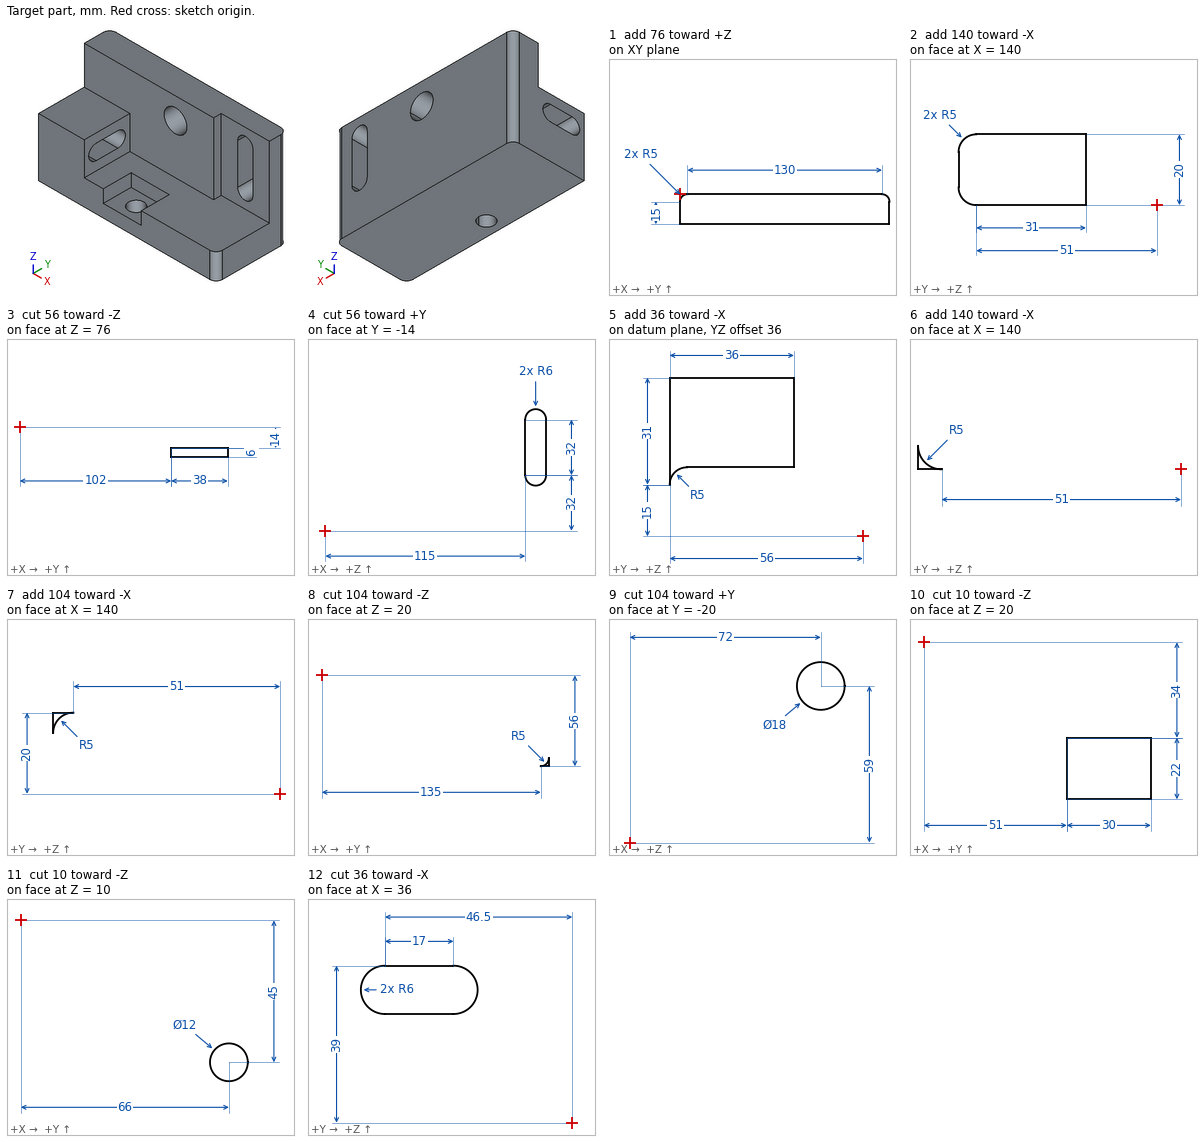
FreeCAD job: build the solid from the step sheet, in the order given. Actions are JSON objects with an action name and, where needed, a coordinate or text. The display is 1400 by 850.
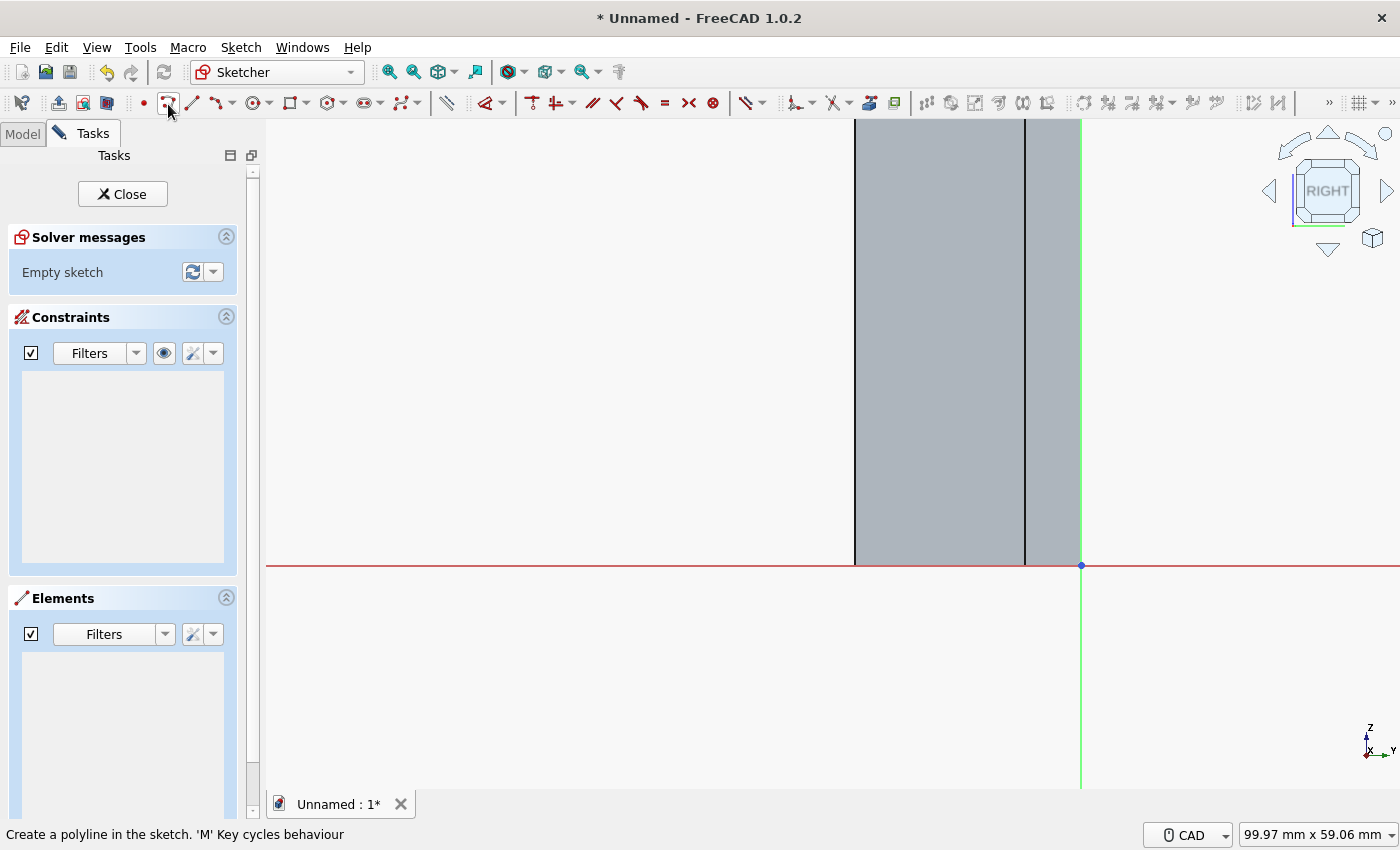
{"action": "left_click", "coordinate": [503, 566]}
{"action": "left_click", "coordinate": [855, 557]}
{"action": "left_click", "coordinate": [855, 339]}
{"action": "left_click", "coordinate": [503, 339]}
{"action": "right_click", "coordinate": [503, 339]}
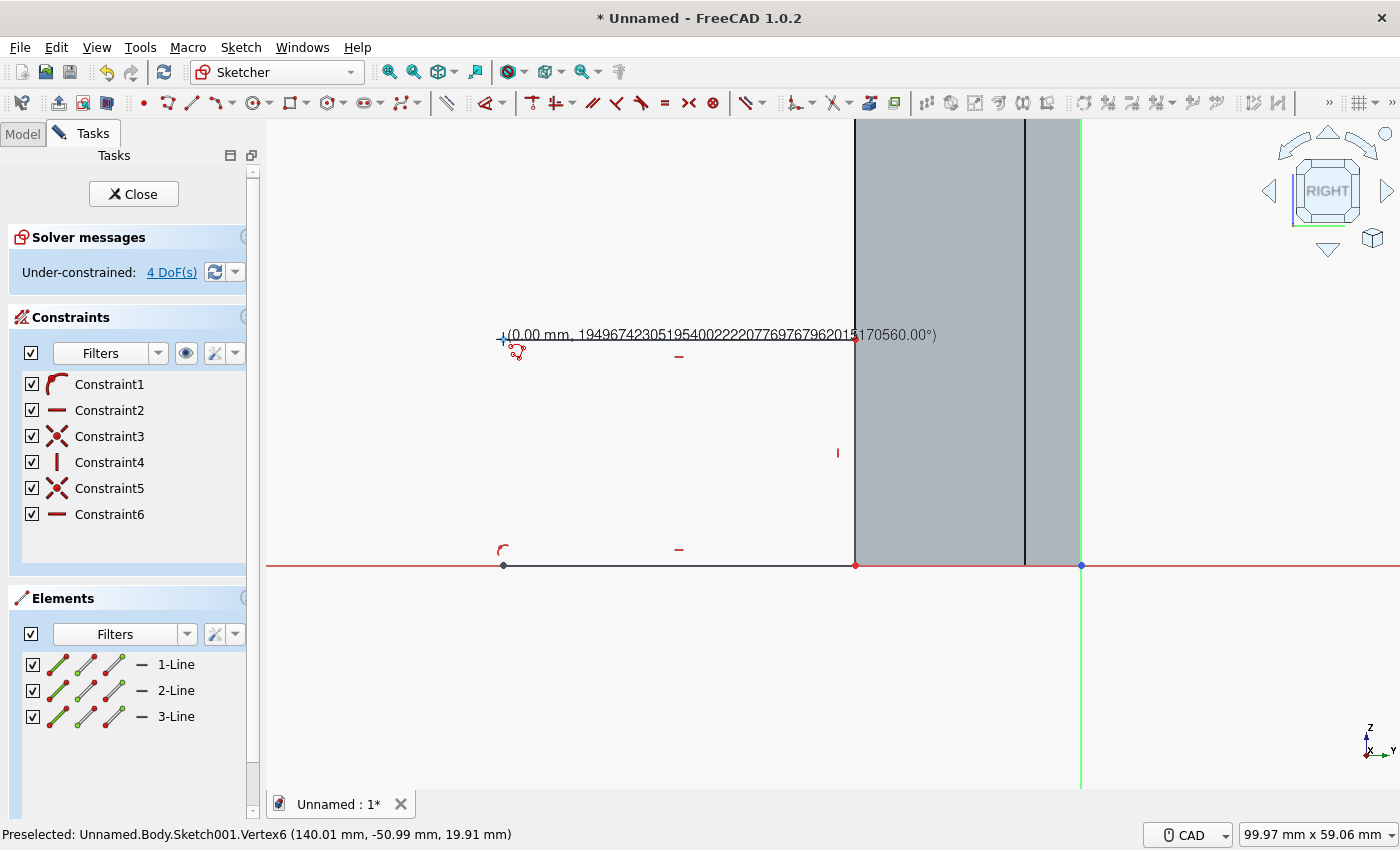
{"action": "key", "text": "g l"}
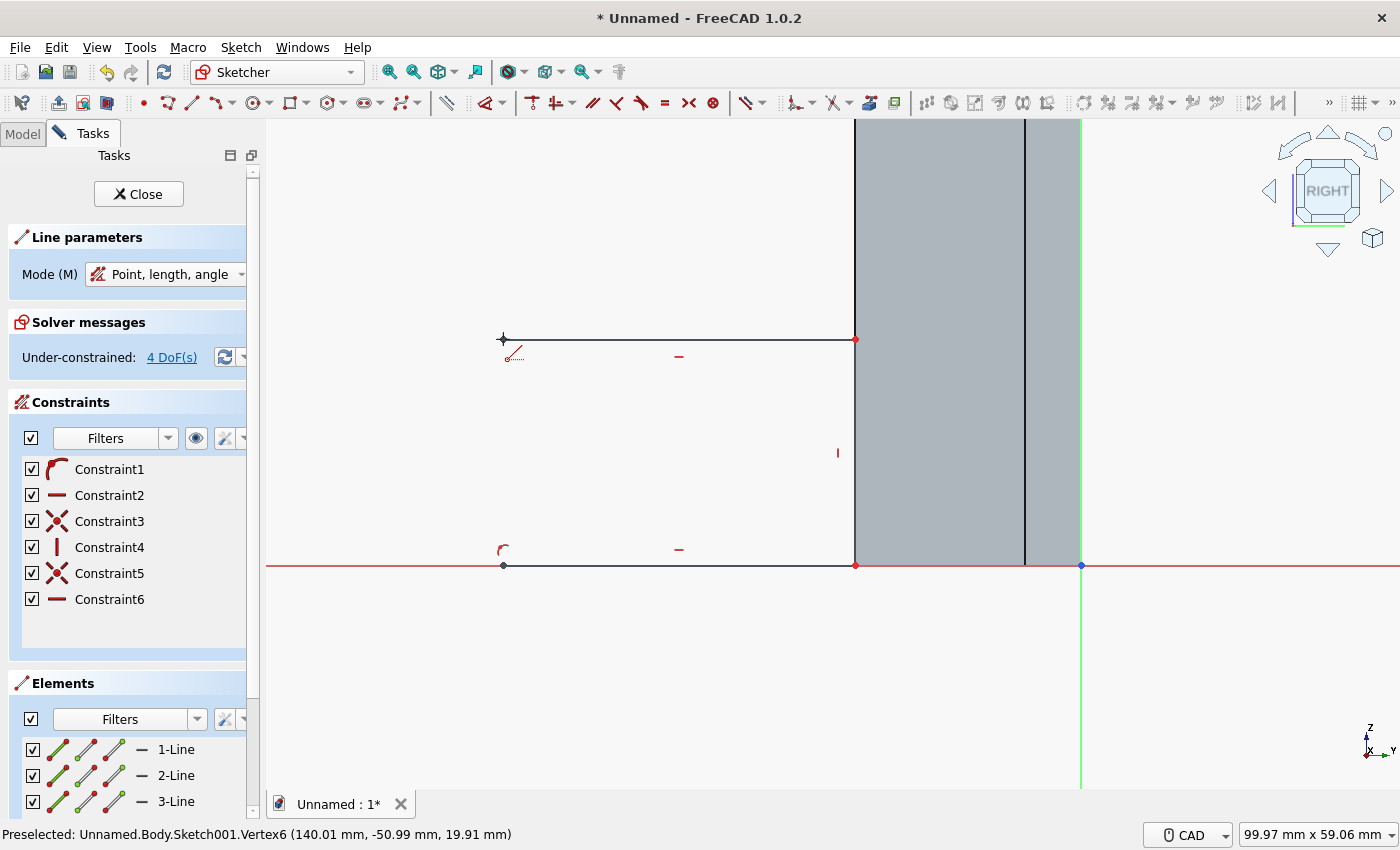
{"action": "left_click", "coordinate": [446, 396]}
{"action": "left_click", "coordinate": [446, 509]}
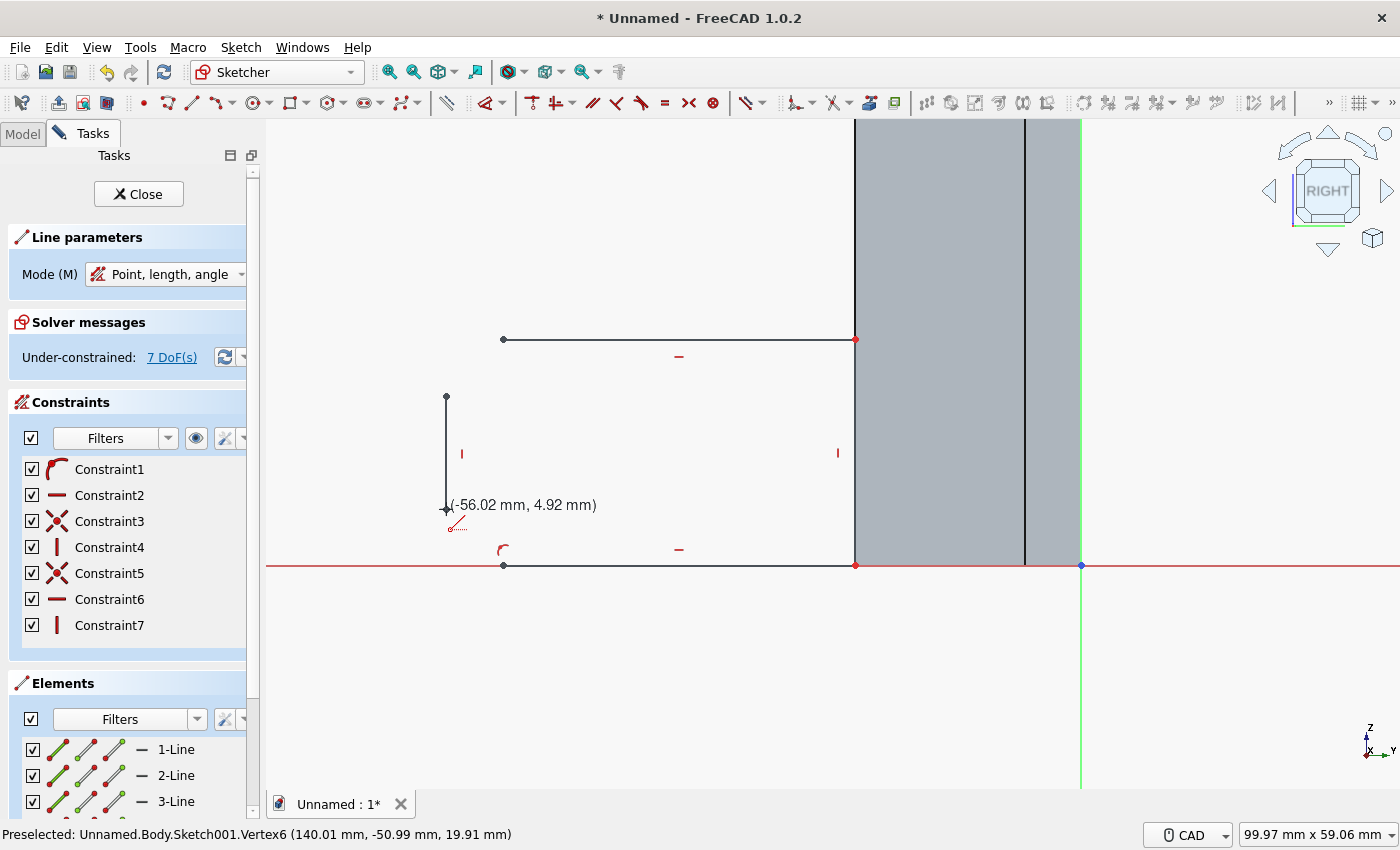
{"action": "left_click", "coordinate": [216, 104]}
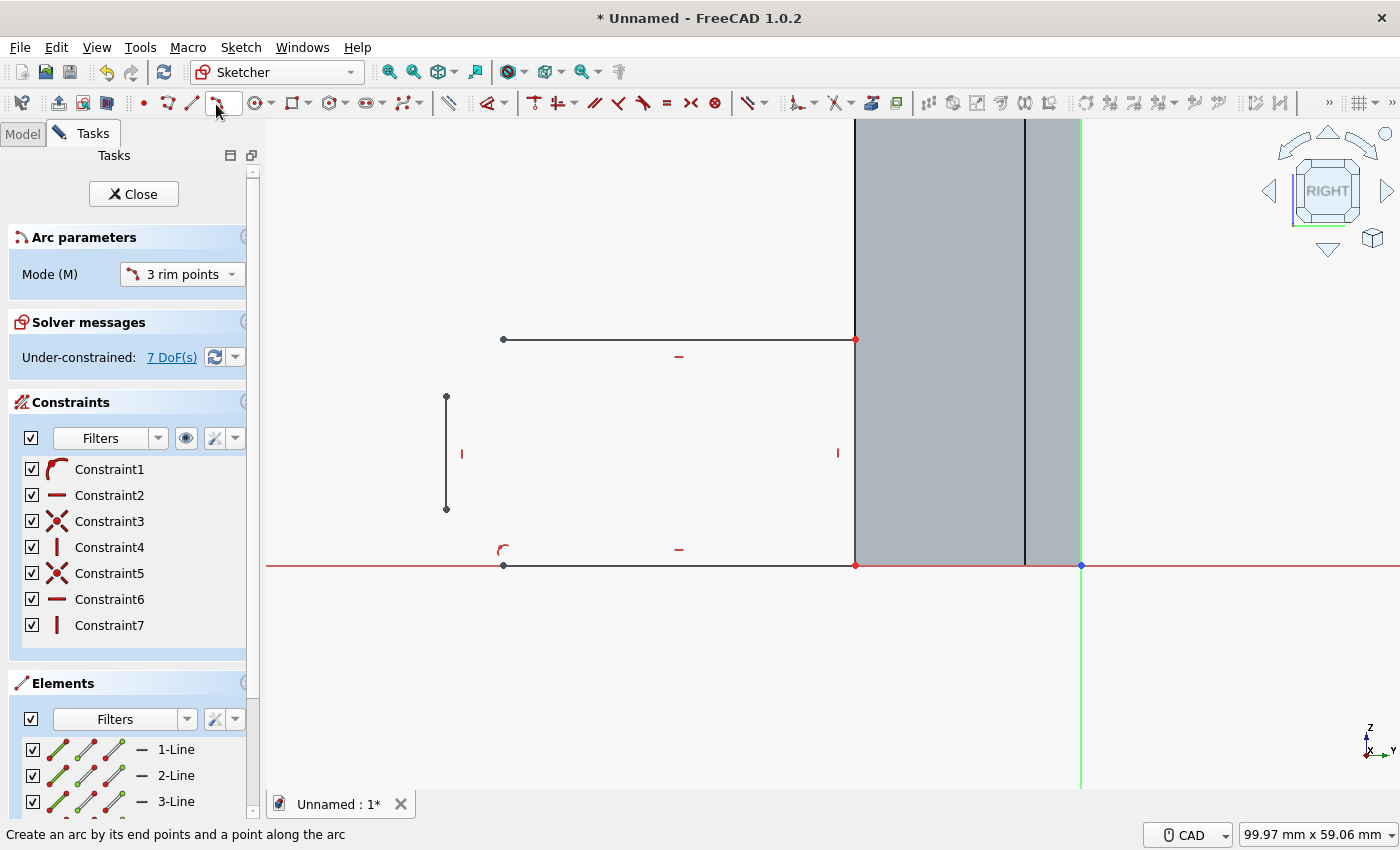
{"action": "left_click", "coordinate": [503, 340]}
{"action": "left_click", "coordinate": [446, 397]}
{"action": "left_click", "coordinate": [463, 356]}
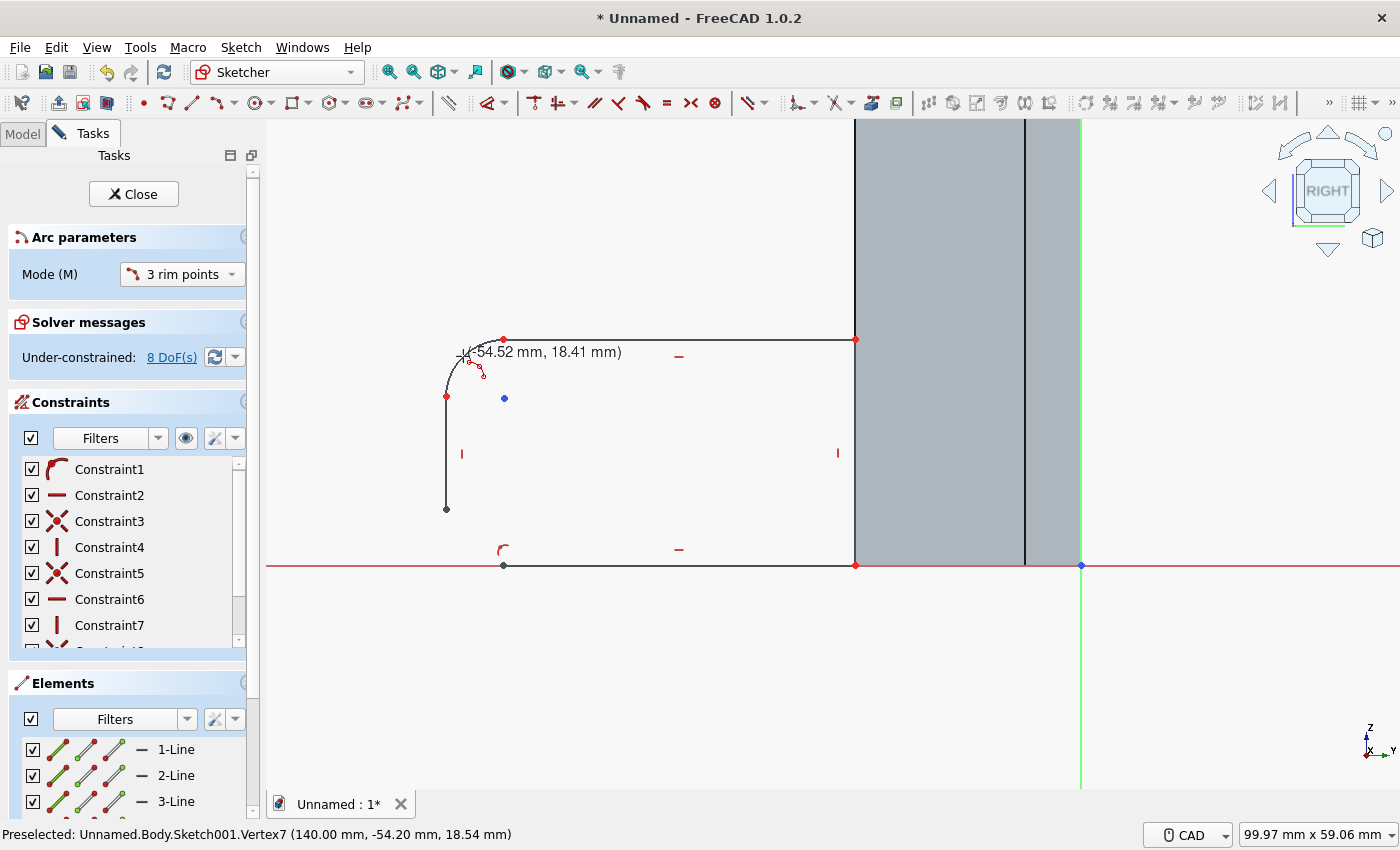
{"action": "left_click", "coordinate": [446, 510]}
{"action": "left_click", "coordinate": [503, 566]}
{"action": "left_click", "coordinate": [463, 549]}
{"action": "key", "text": "Escape"}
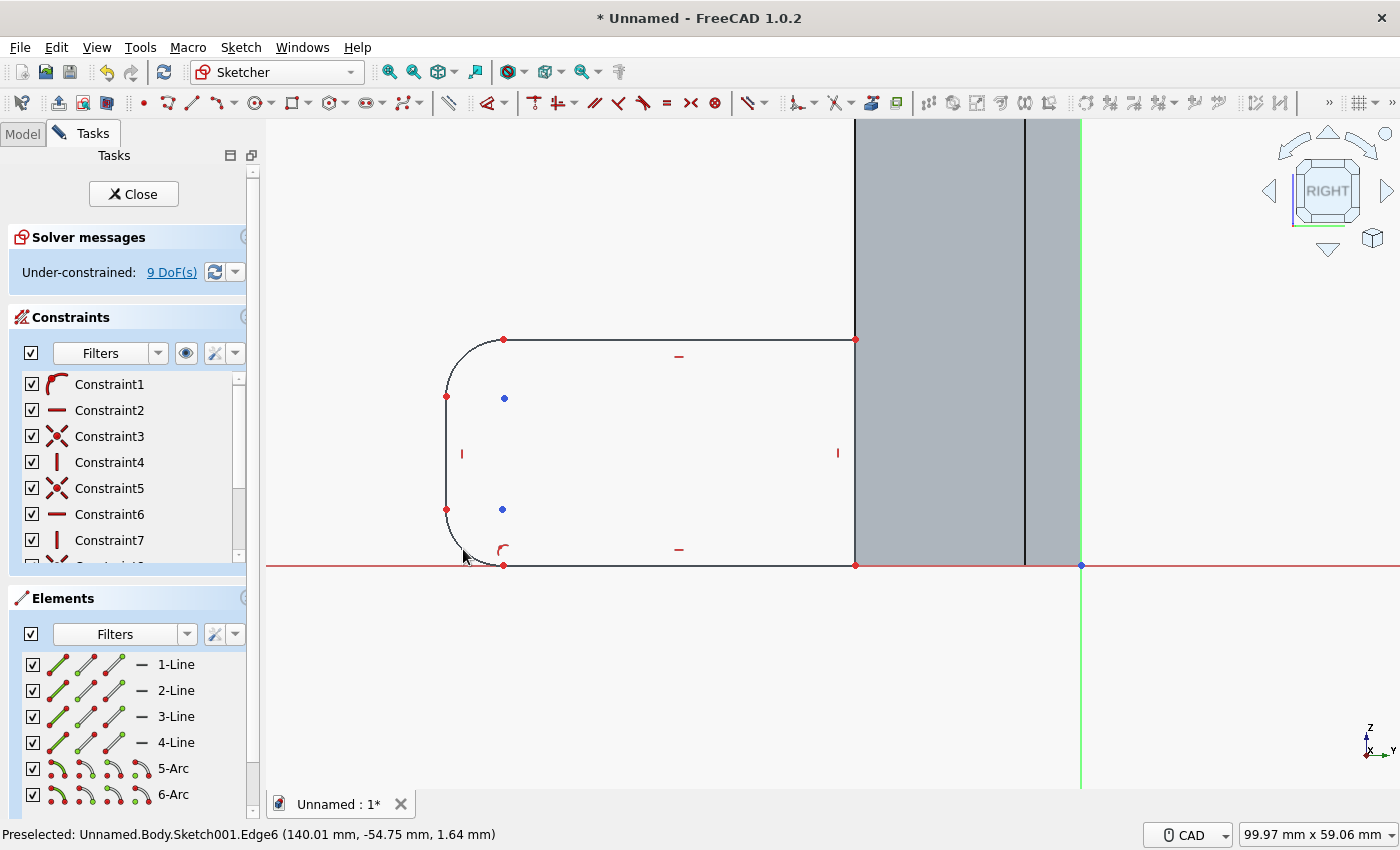
{"action": "left_click", "coordinate": [609, 566]}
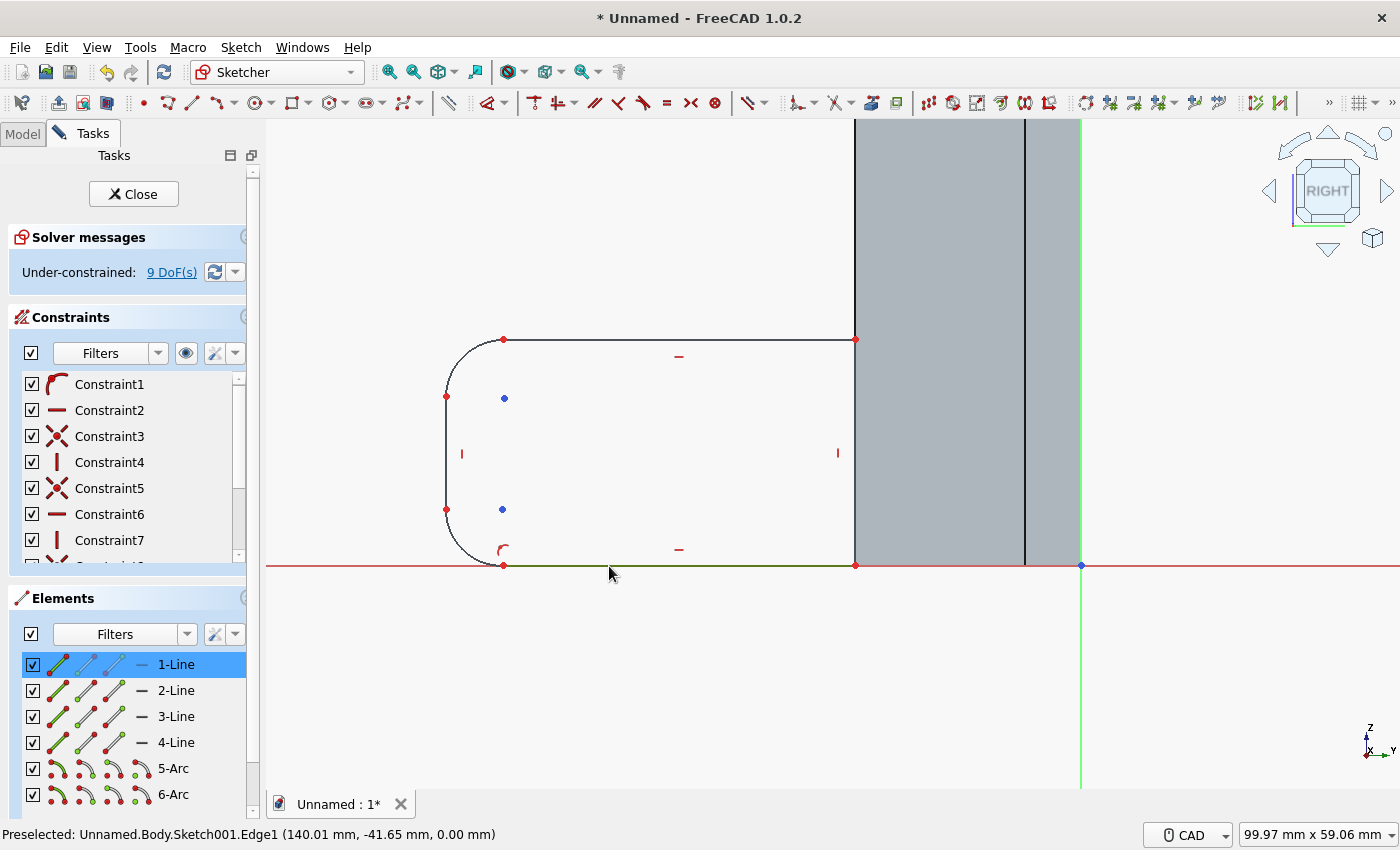
{"action": "left_click", "coordinate": [452, 536]}